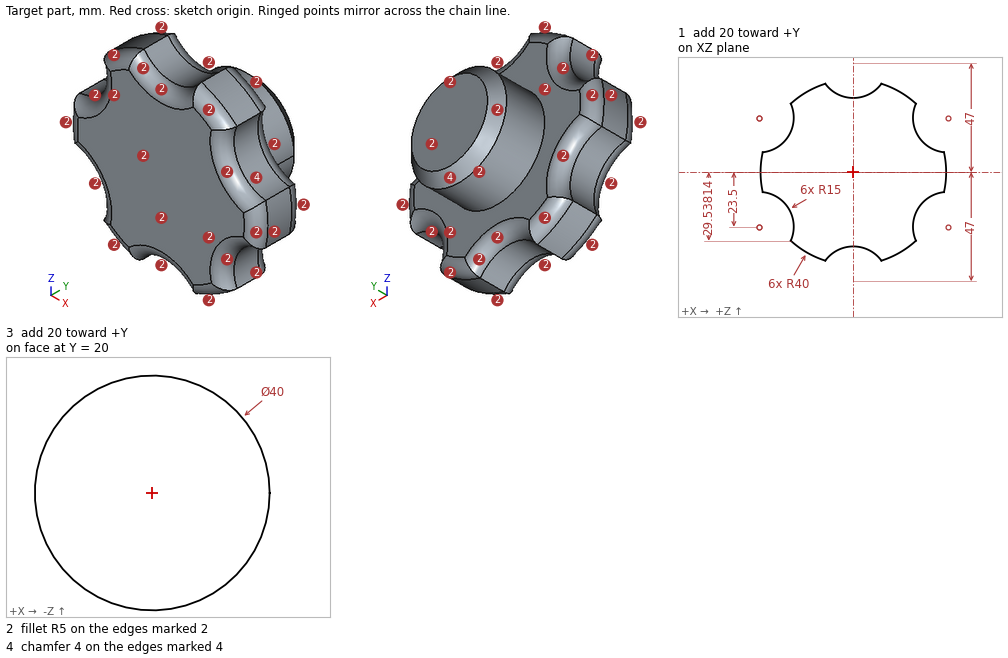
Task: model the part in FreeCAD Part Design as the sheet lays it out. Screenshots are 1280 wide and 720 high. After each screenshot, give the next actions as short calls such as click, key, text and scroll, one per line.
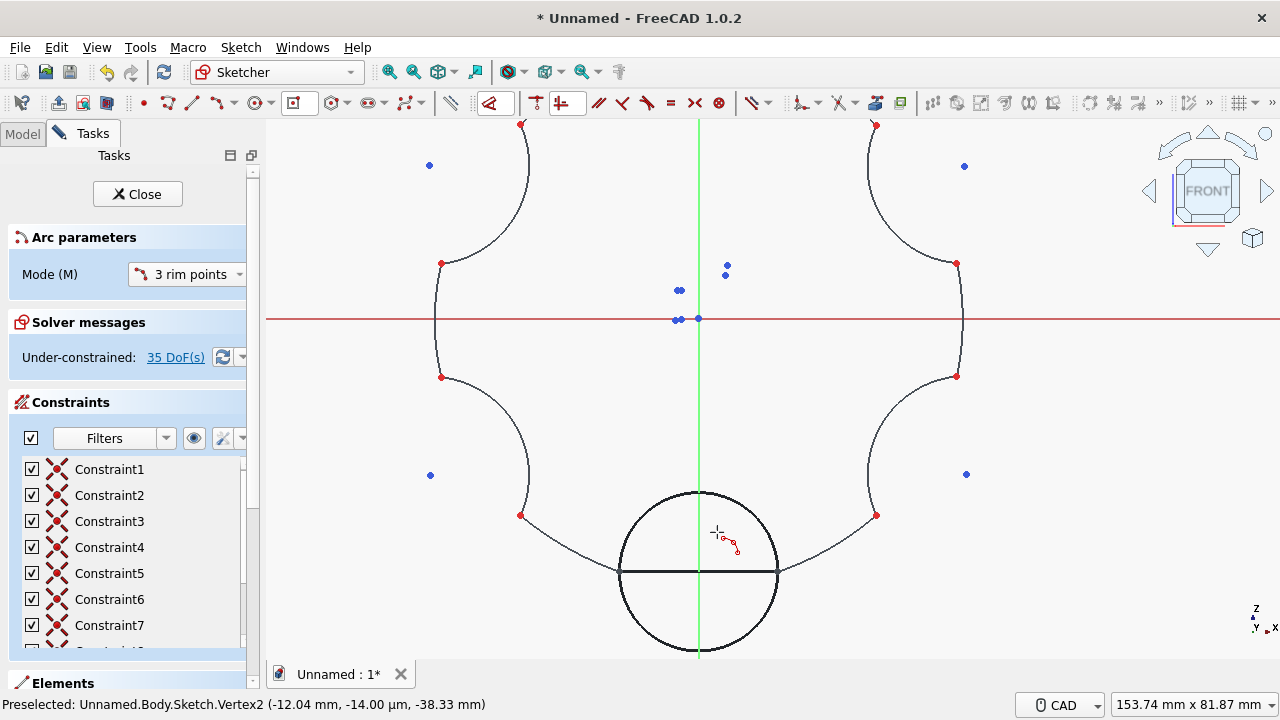
click(717, 532)
key(Escape)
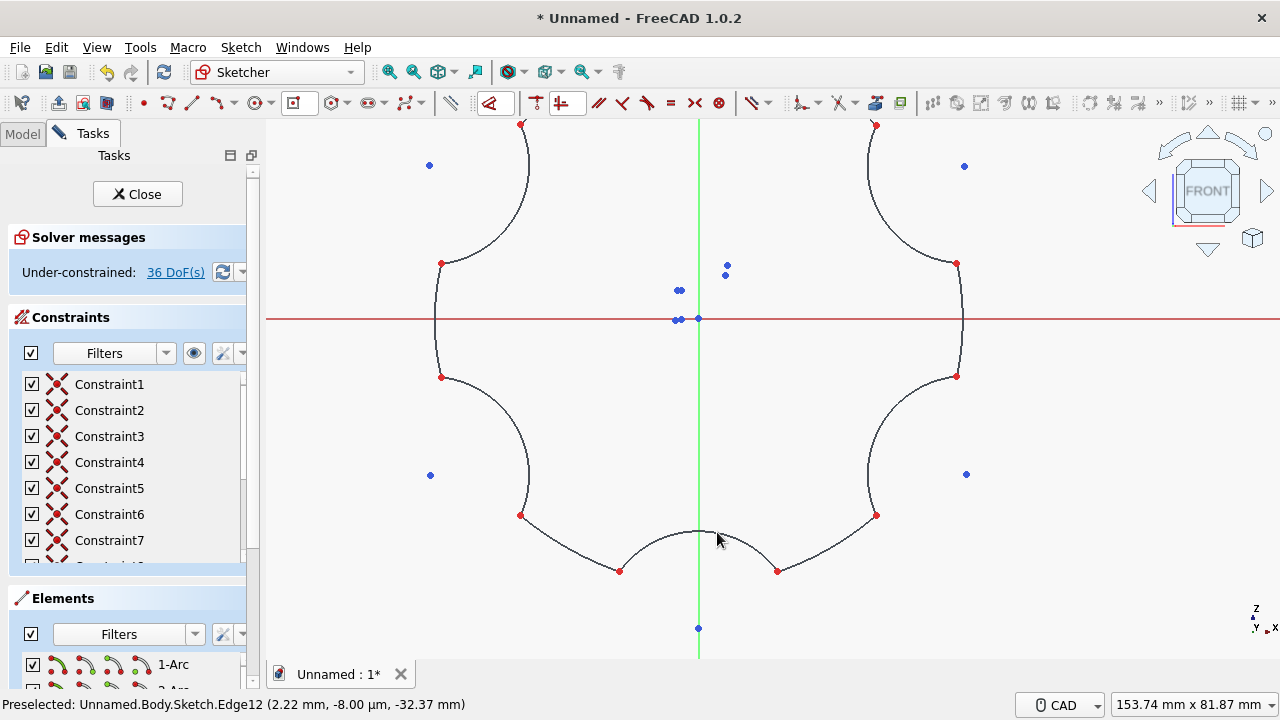
click(548, 536)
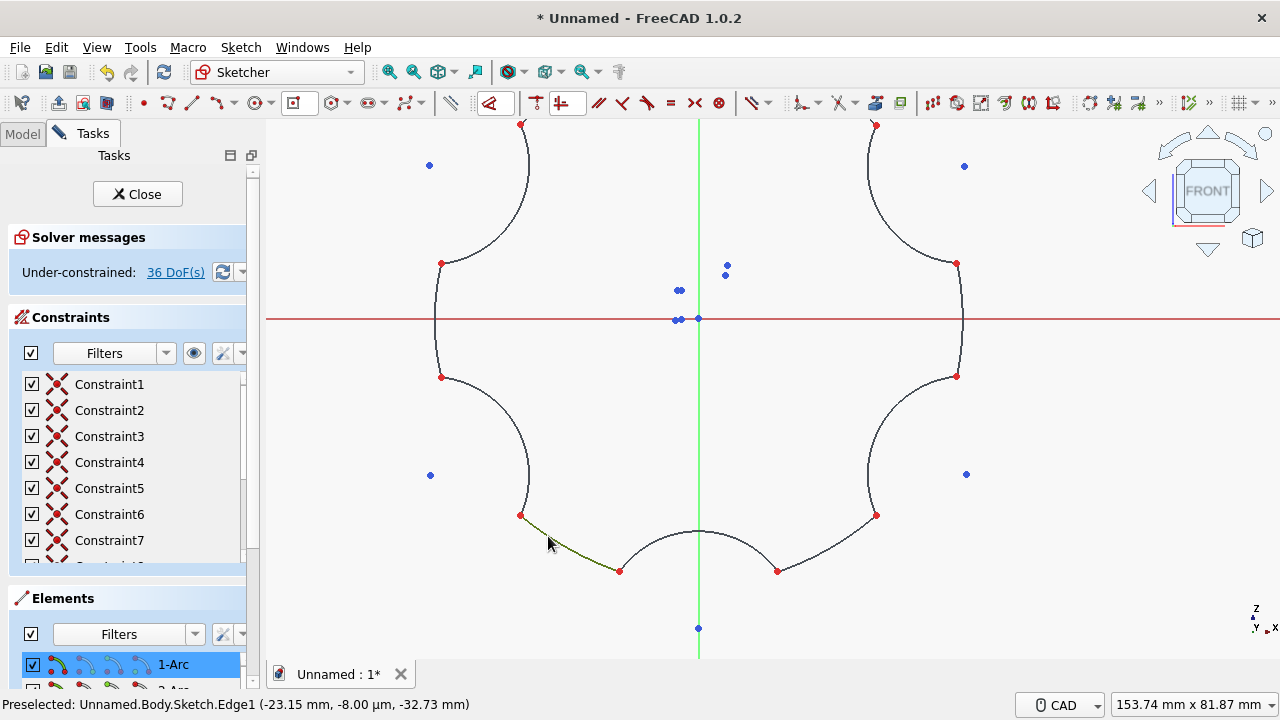
click(436, 298)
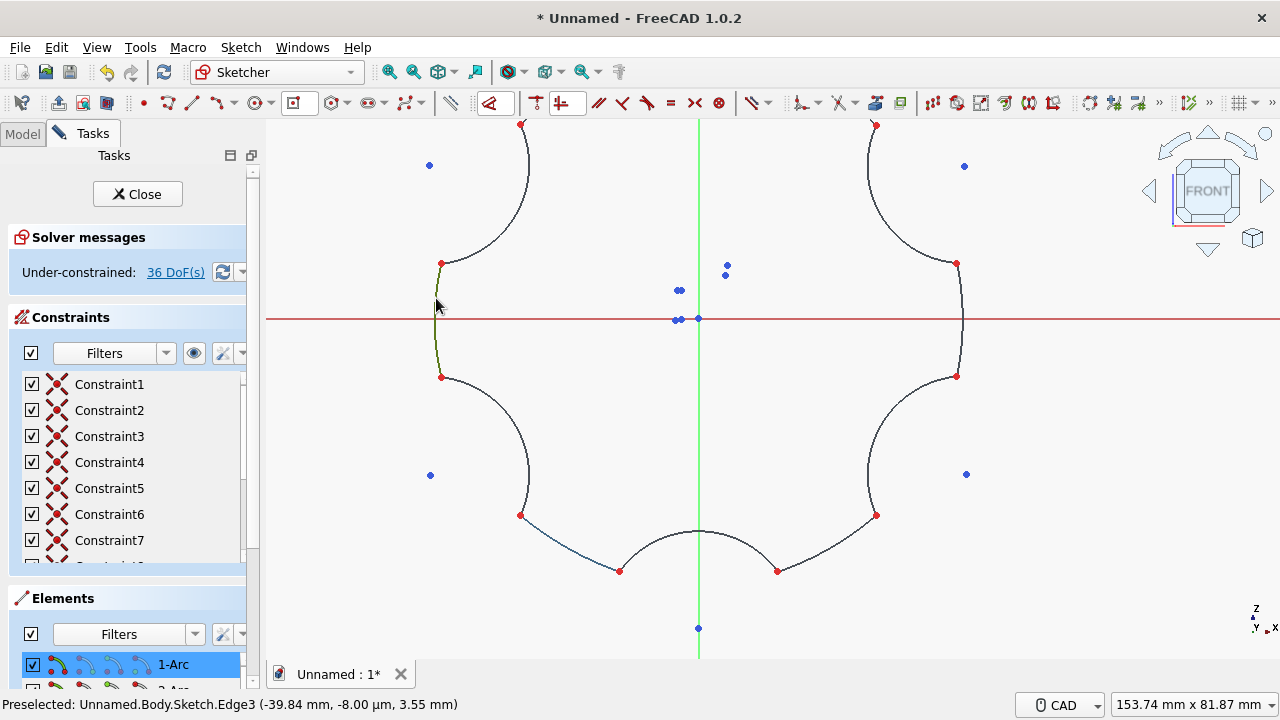
key(c)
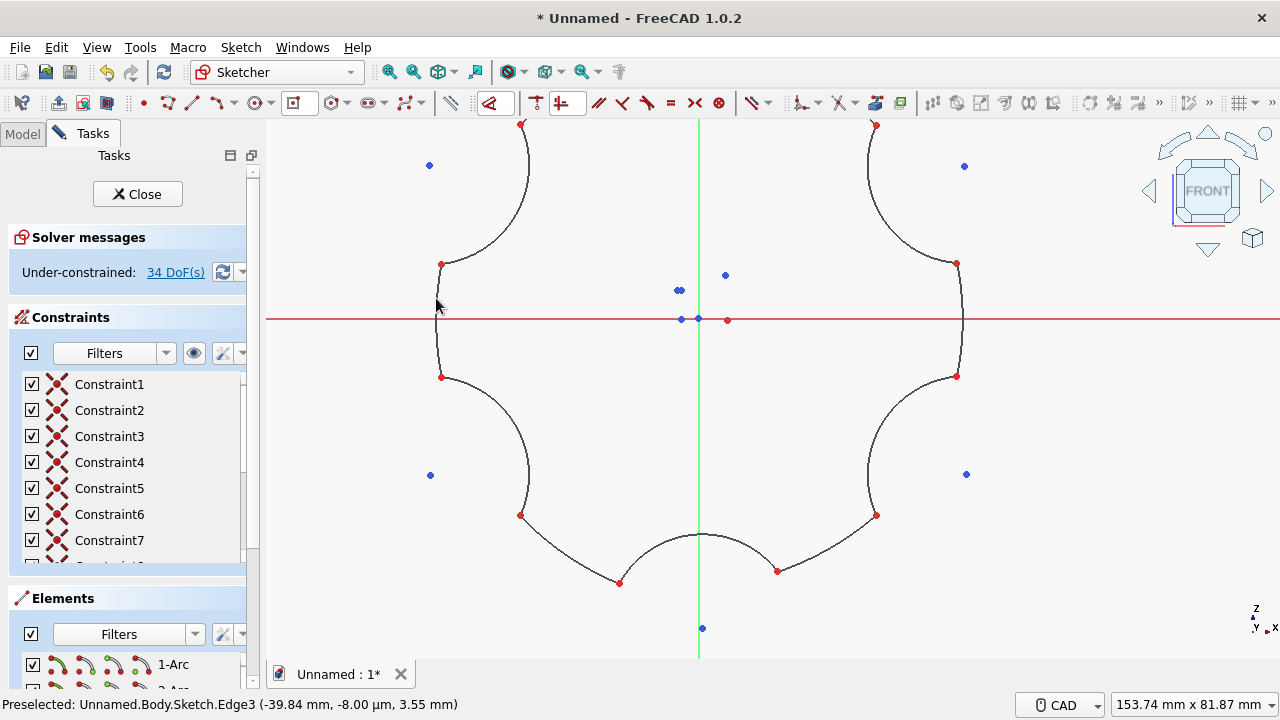
click(547, 540)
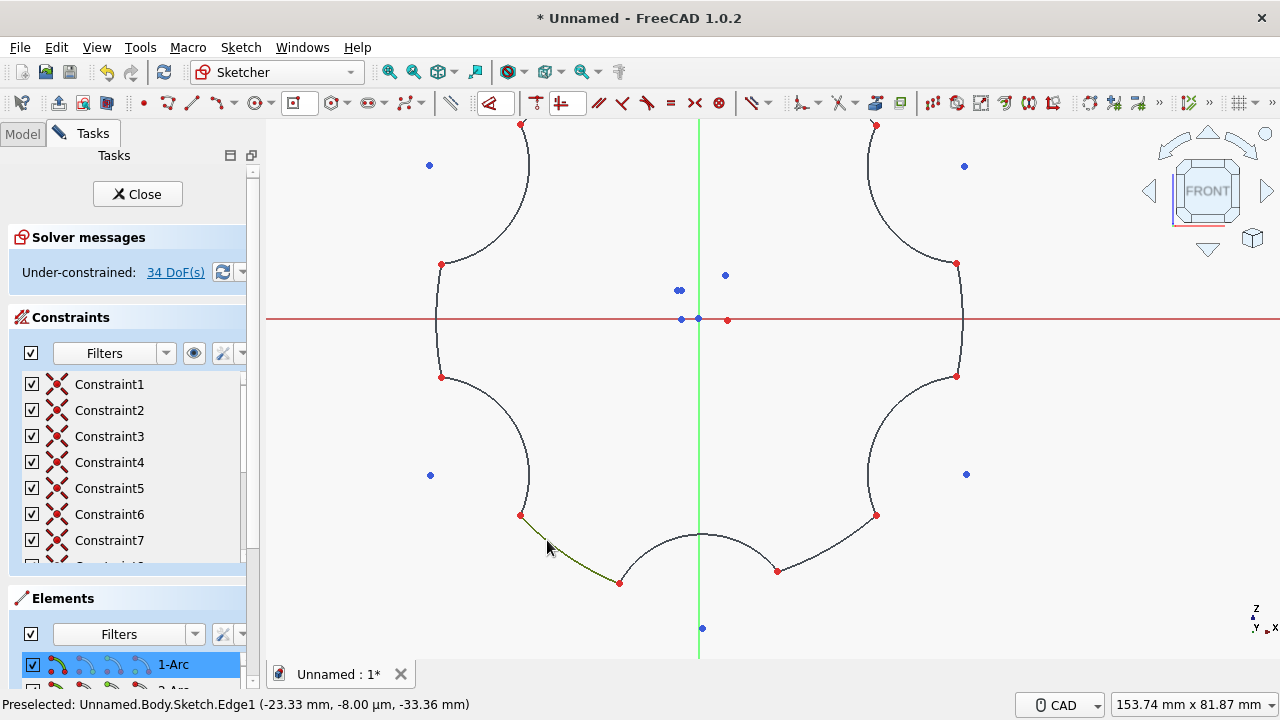
scroll(716, 532, down, 2)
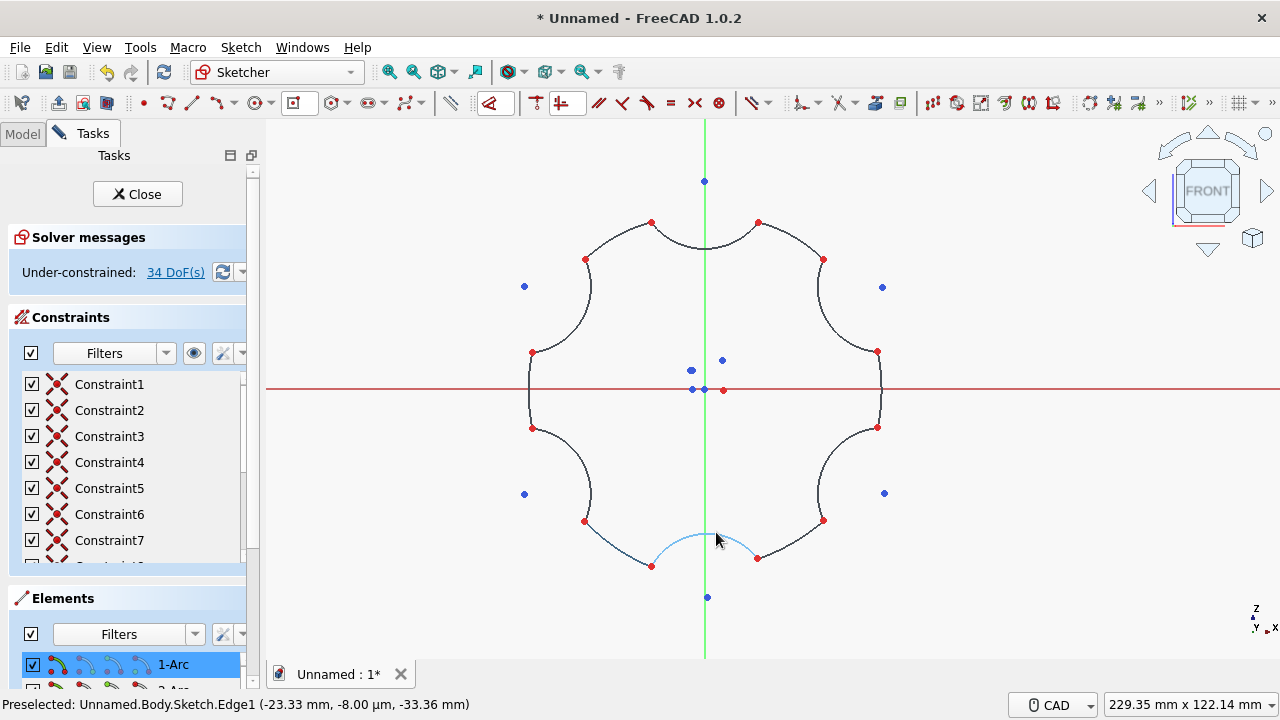
click(630, 230)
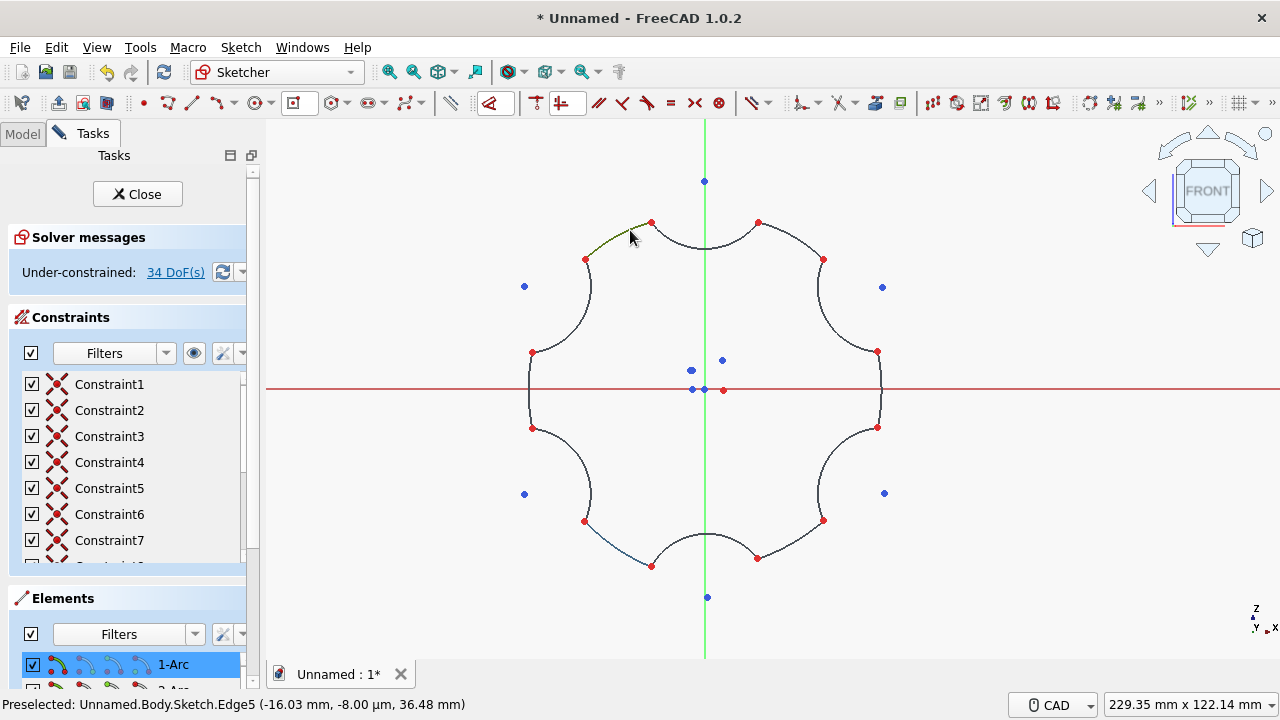
key(c)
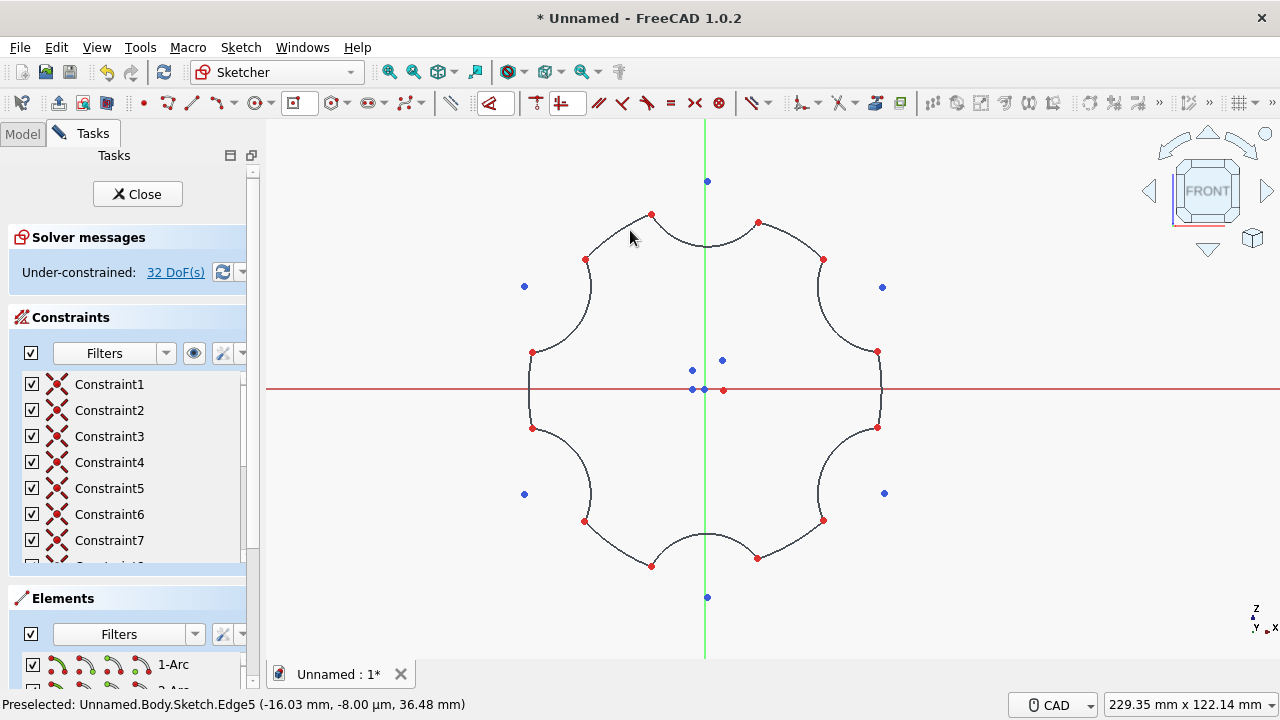
click(603, 538)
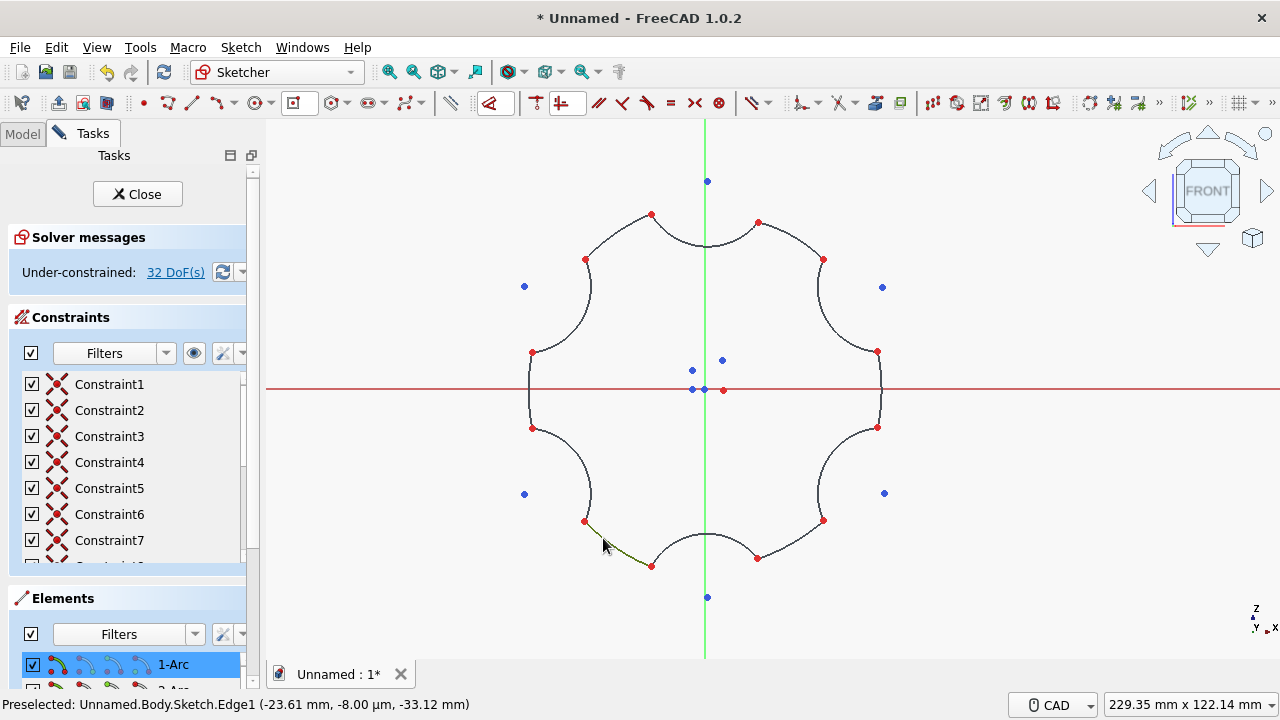
click(806, 245)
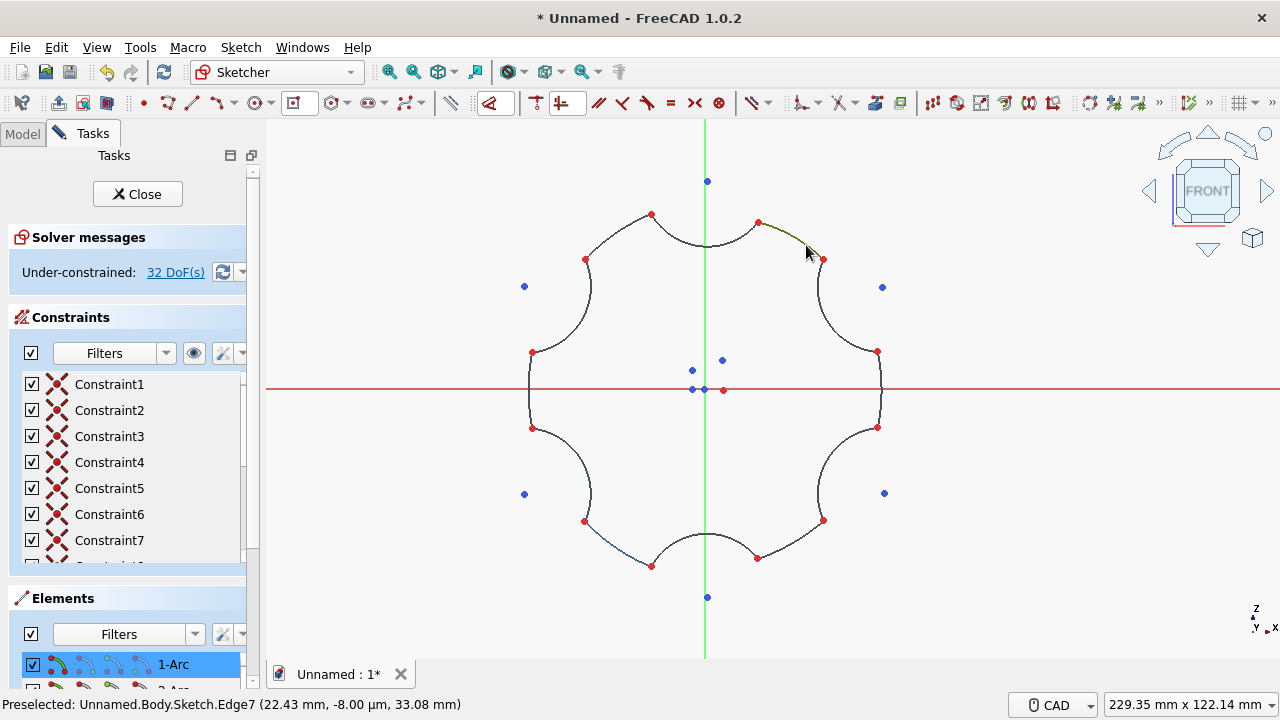
click(536, 104)